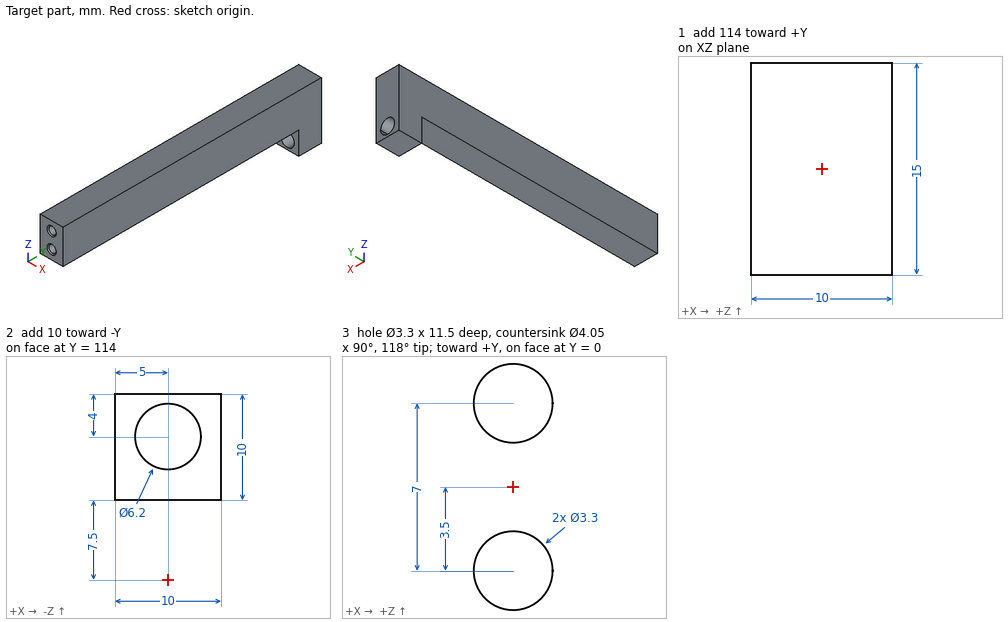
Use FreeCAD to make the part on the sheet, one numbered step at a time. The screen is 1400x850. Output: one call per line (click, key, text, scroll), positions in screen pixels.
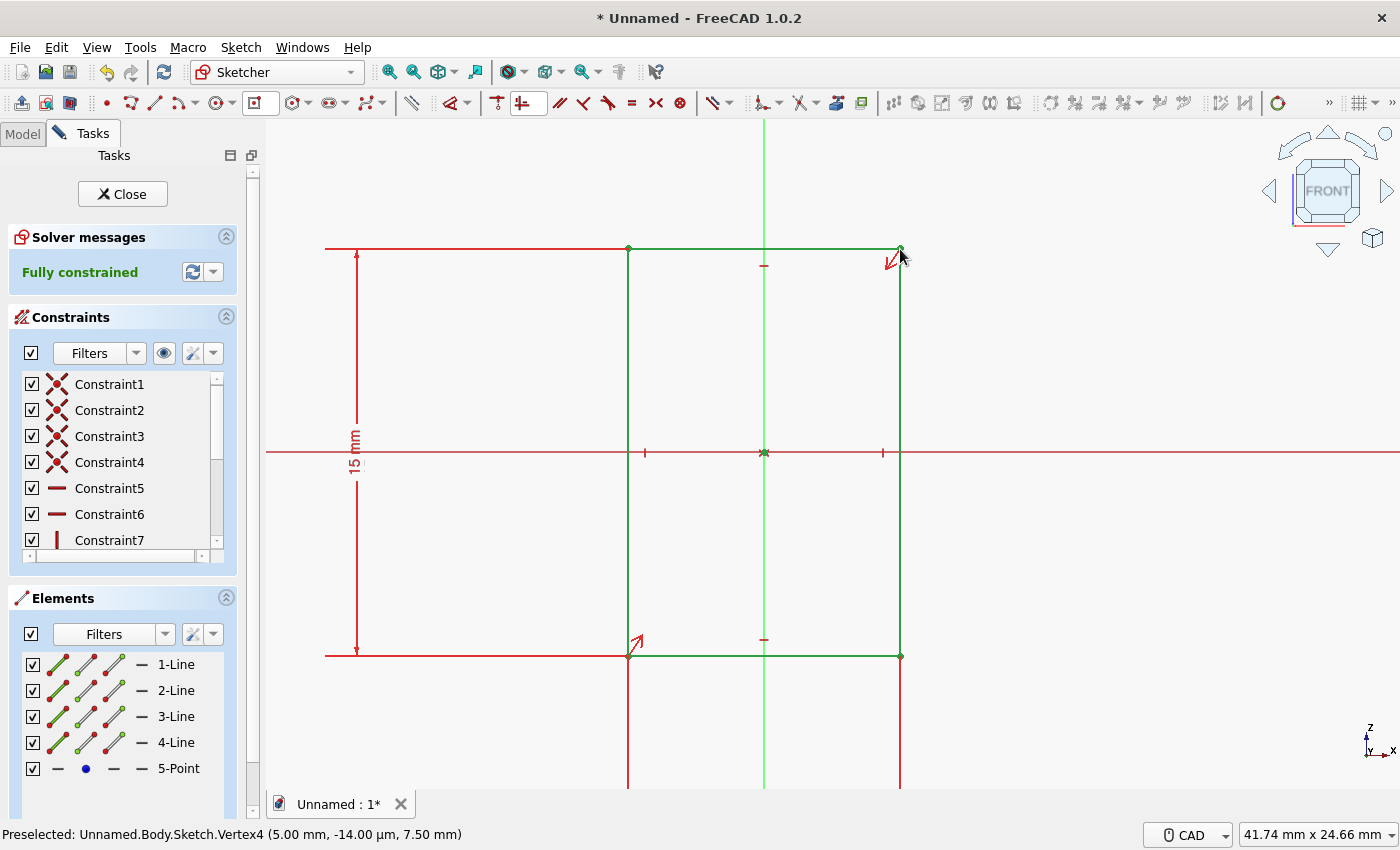
click(123, 194)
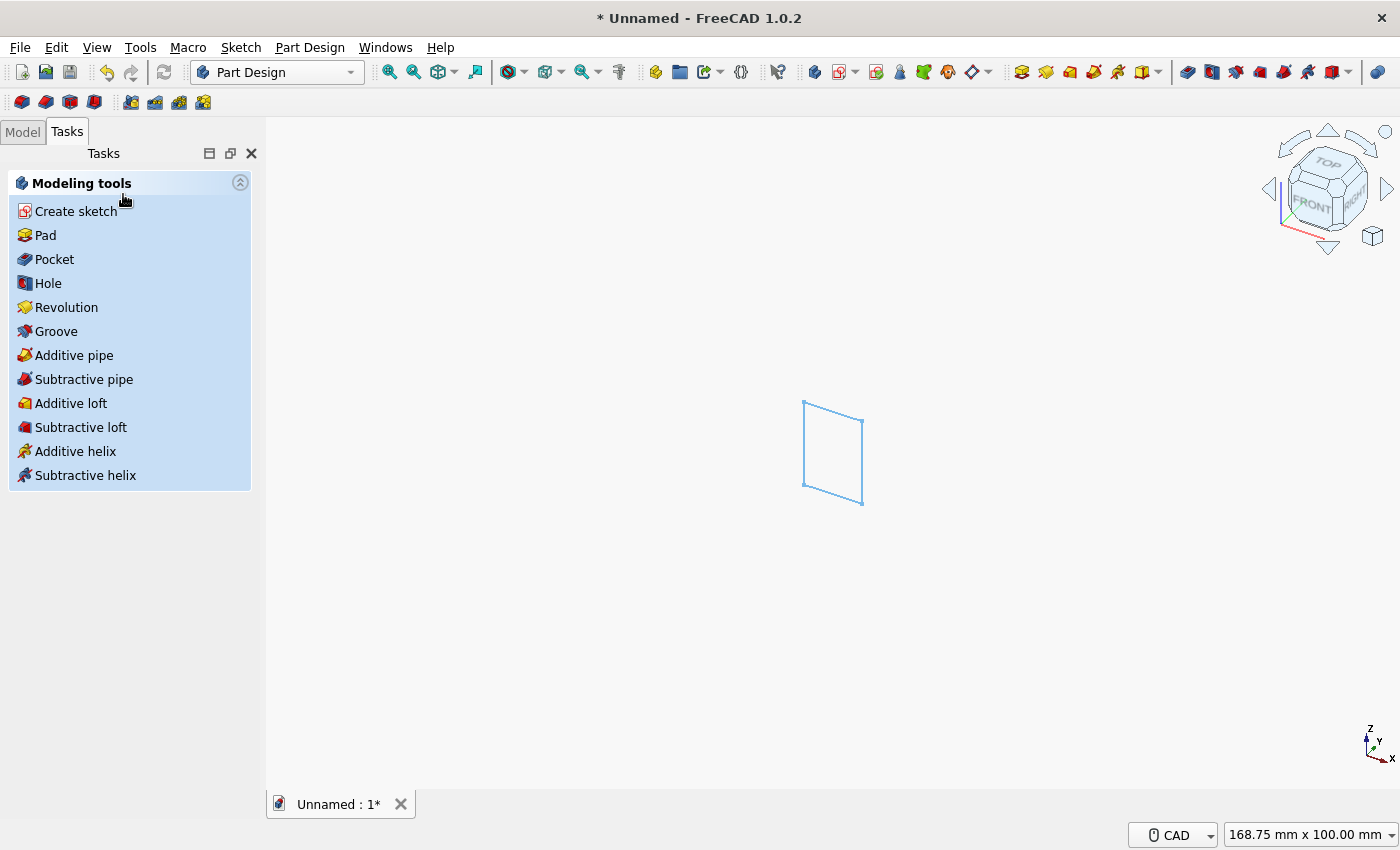
click(1022, 72)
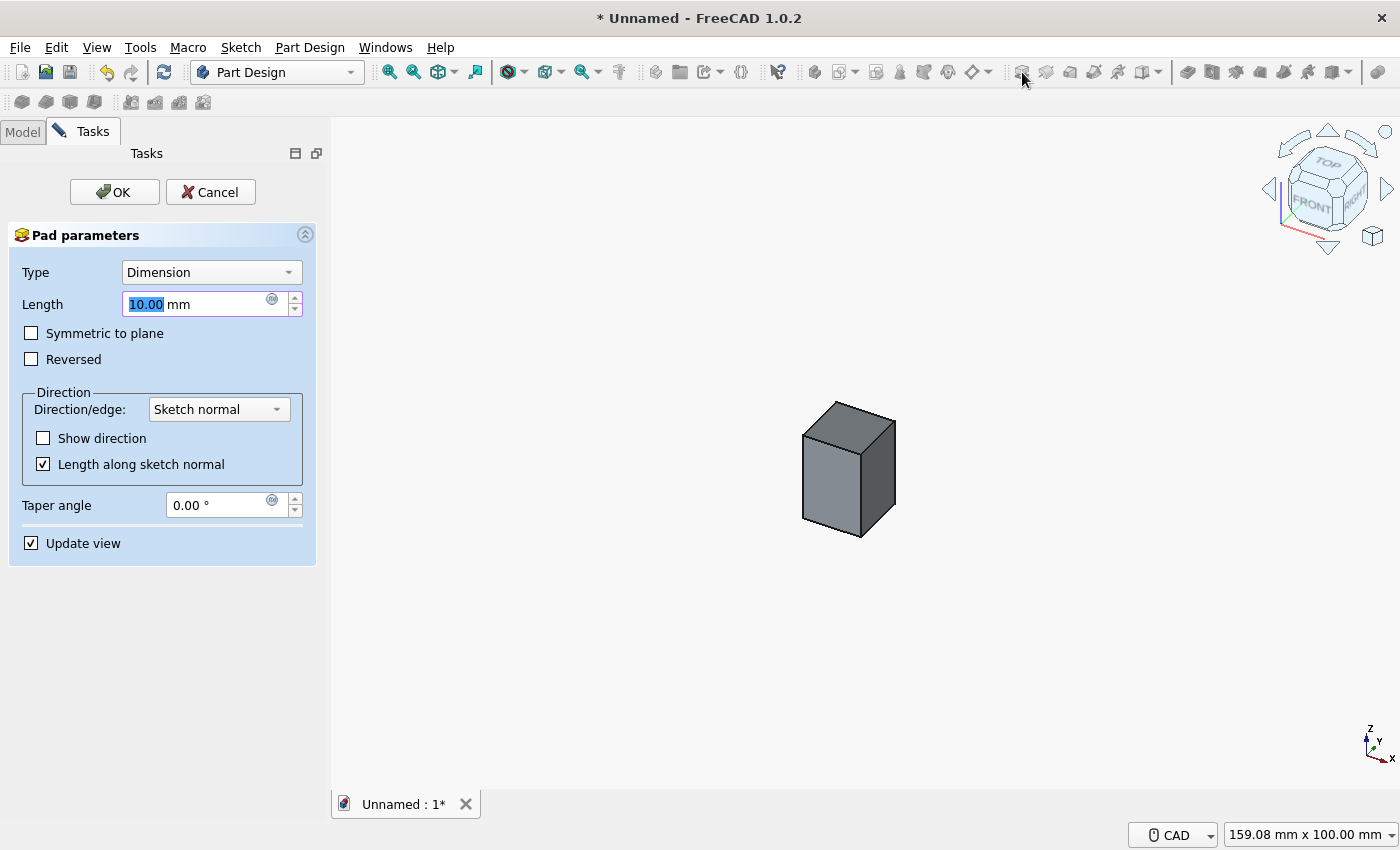
text(114)
key(Tab)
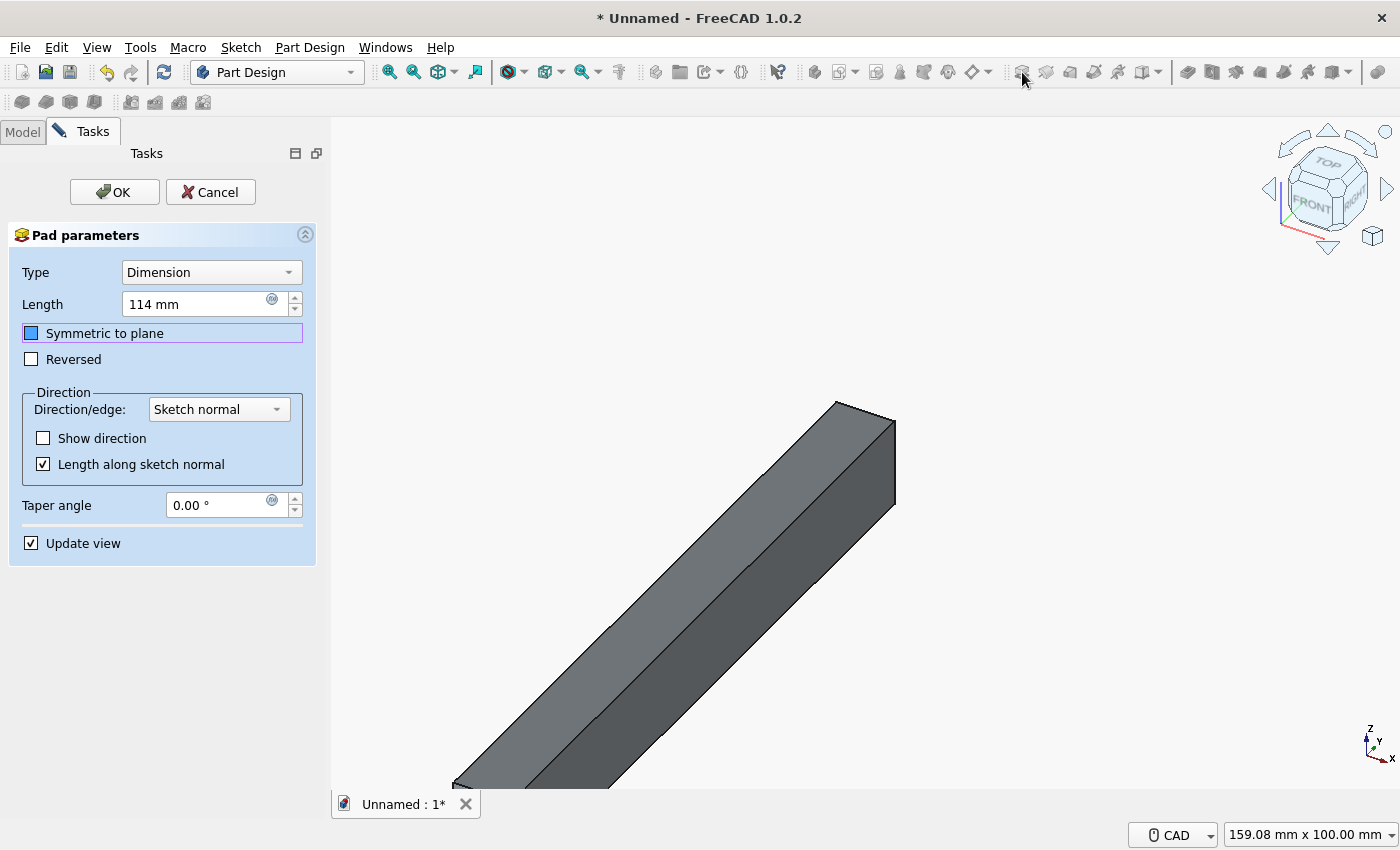
click(30, 359)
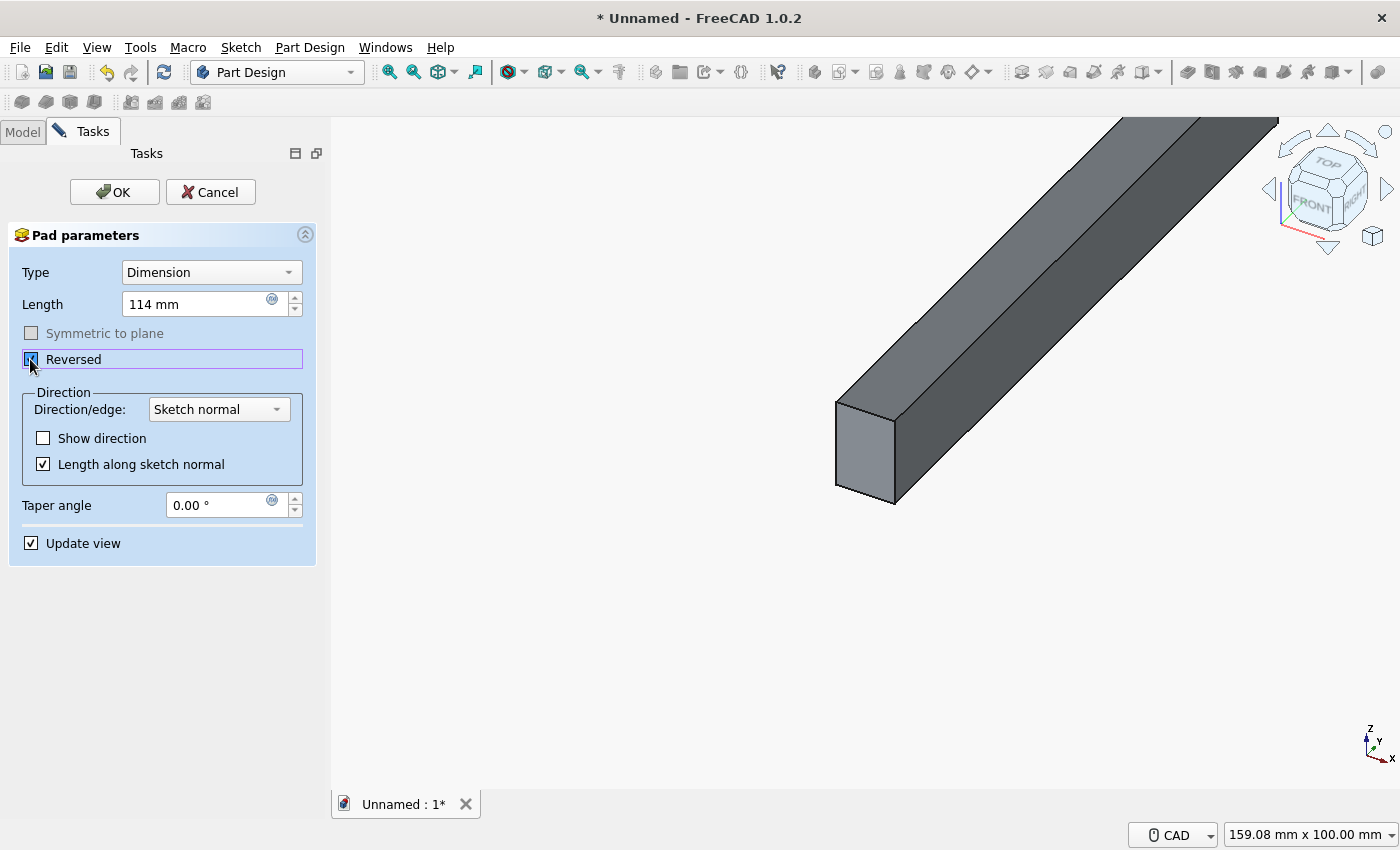
click(115, 192)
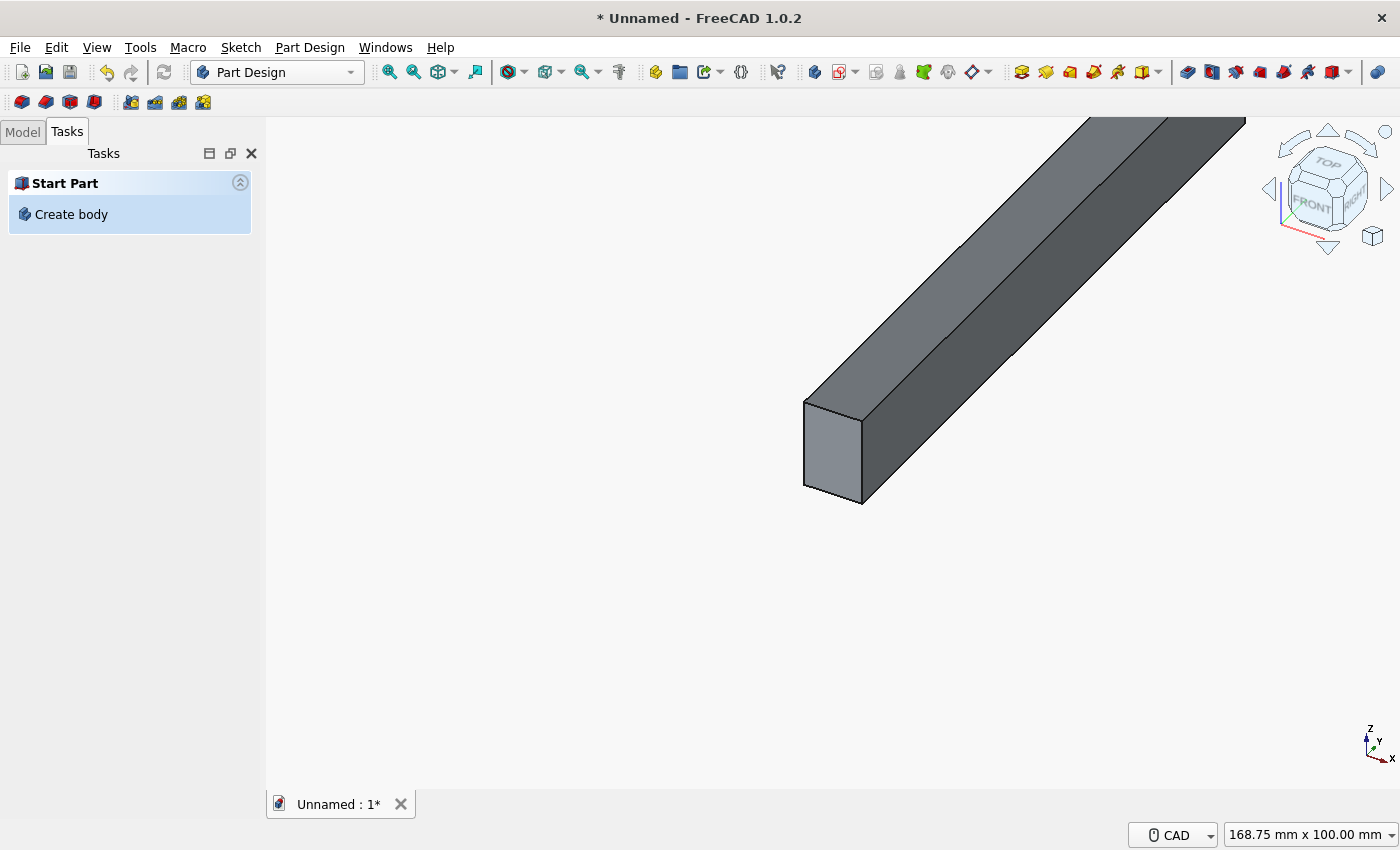
click(390, 72)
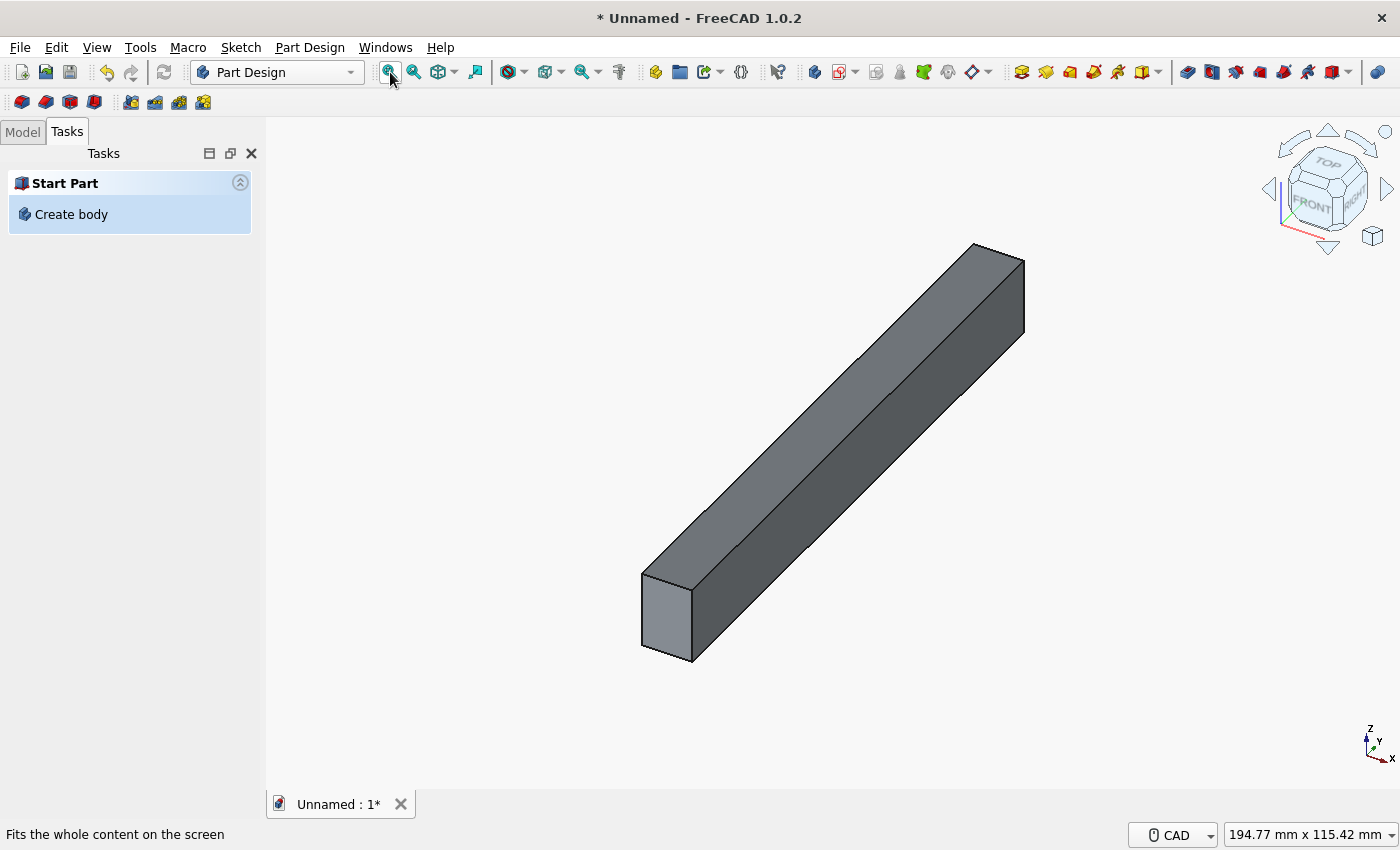
key(4)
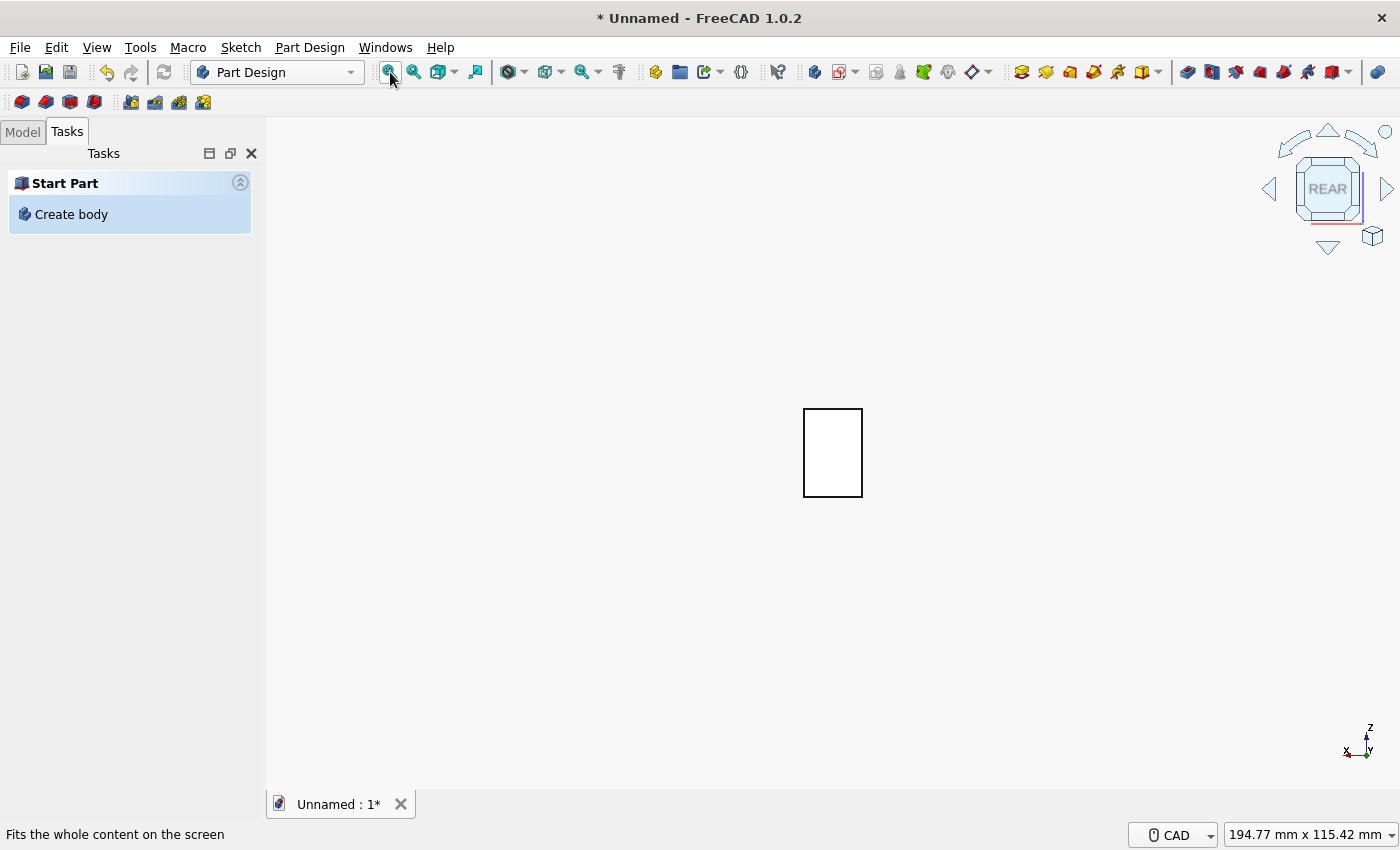
click(390, 72)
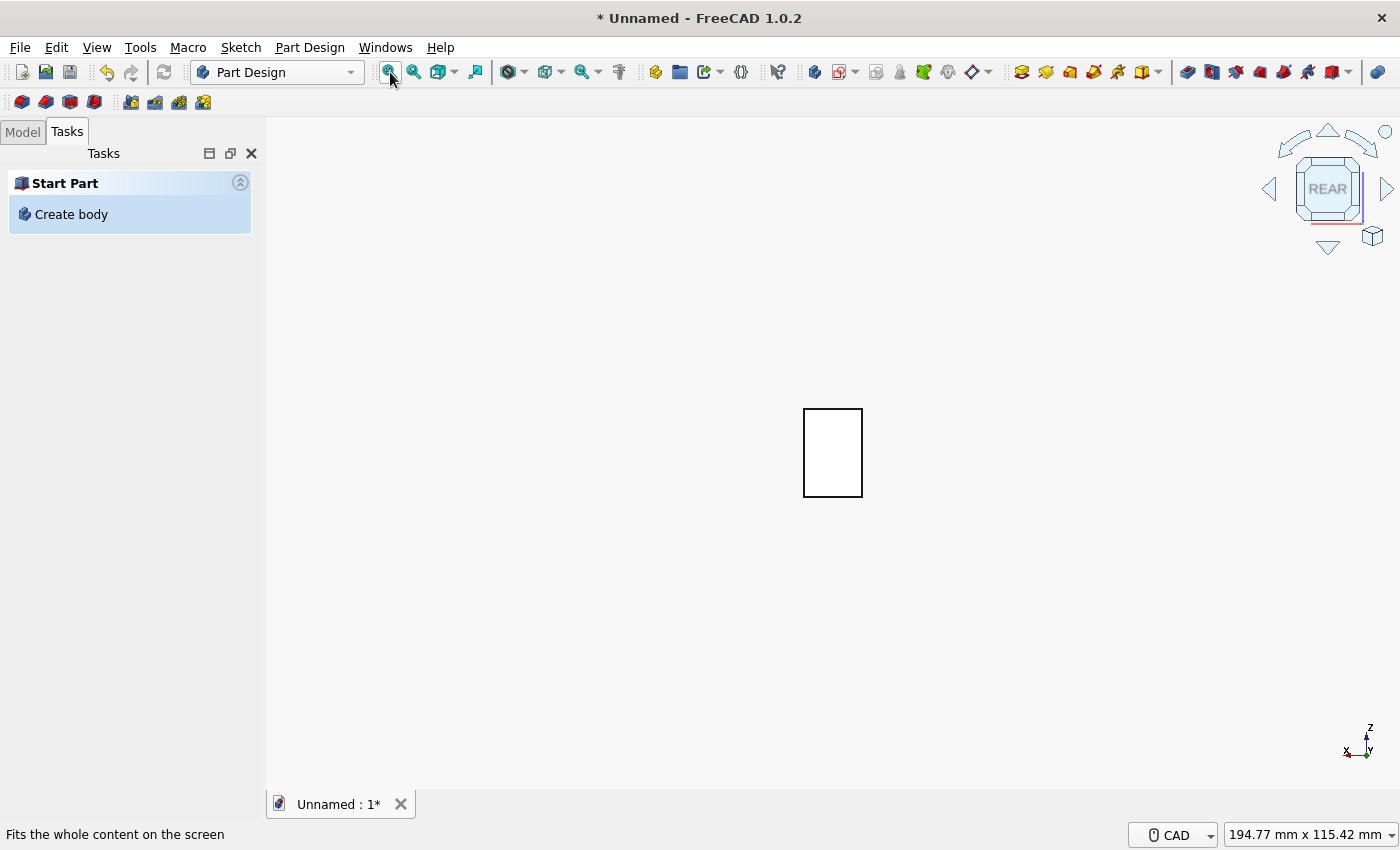
click(833, 440)